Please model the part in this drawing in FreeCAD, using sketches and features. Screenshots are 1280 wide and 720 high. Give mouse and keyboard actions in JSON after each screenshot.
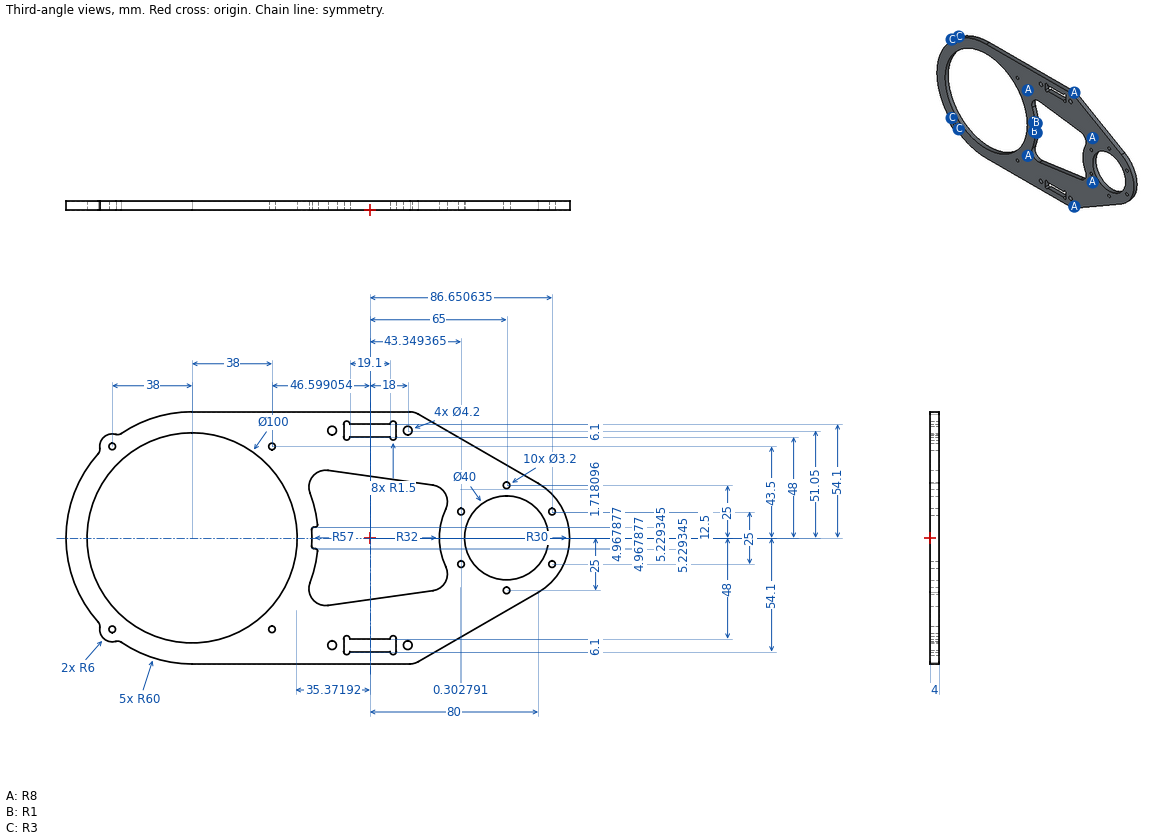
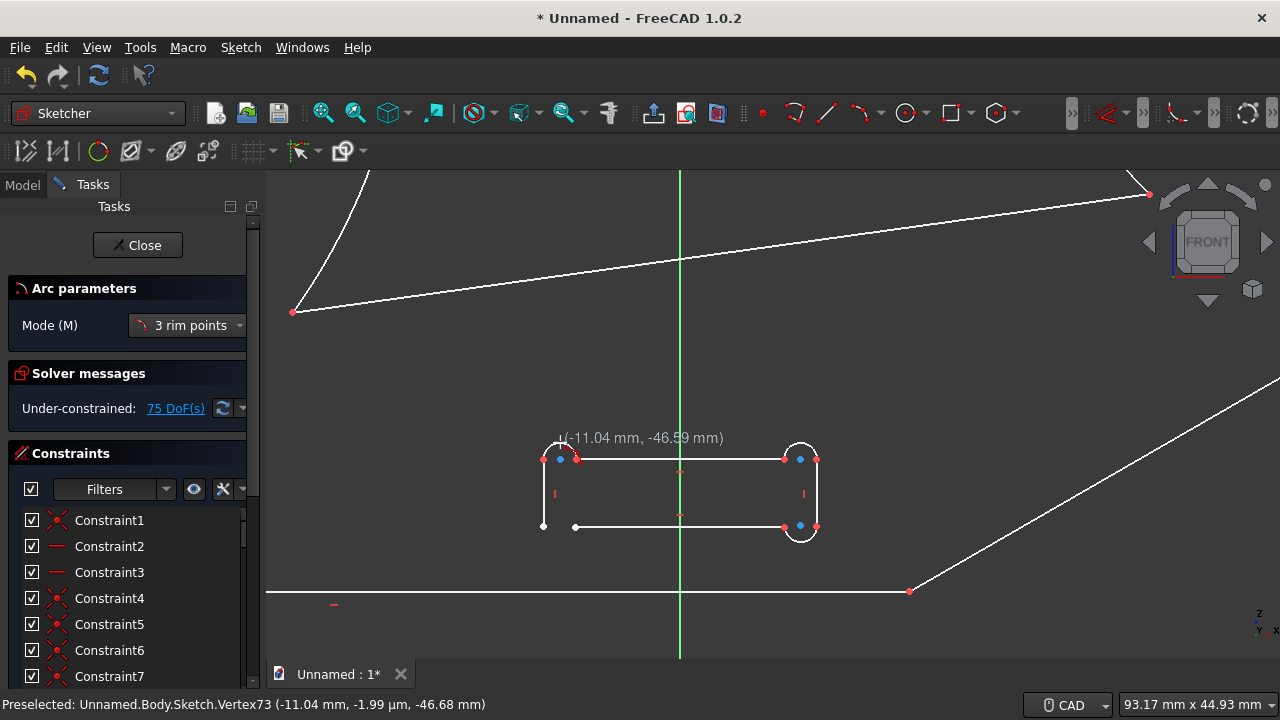
{"action": "left_click", "coordinate": [544, 527]}
{"action": "left_click", "coordinate": [576, 527]}
{"action": "left_click", "coordinate": [560, 541]}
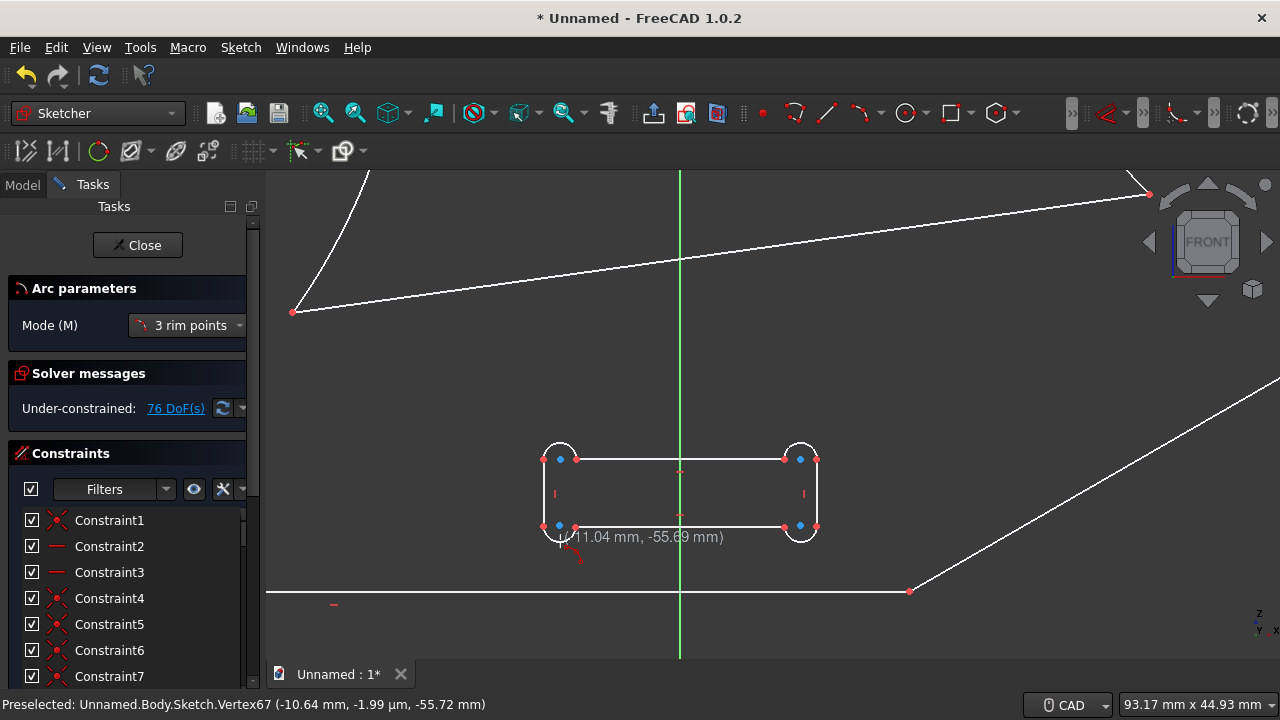
{"action": "left_click", "coordinate": [906, 114]}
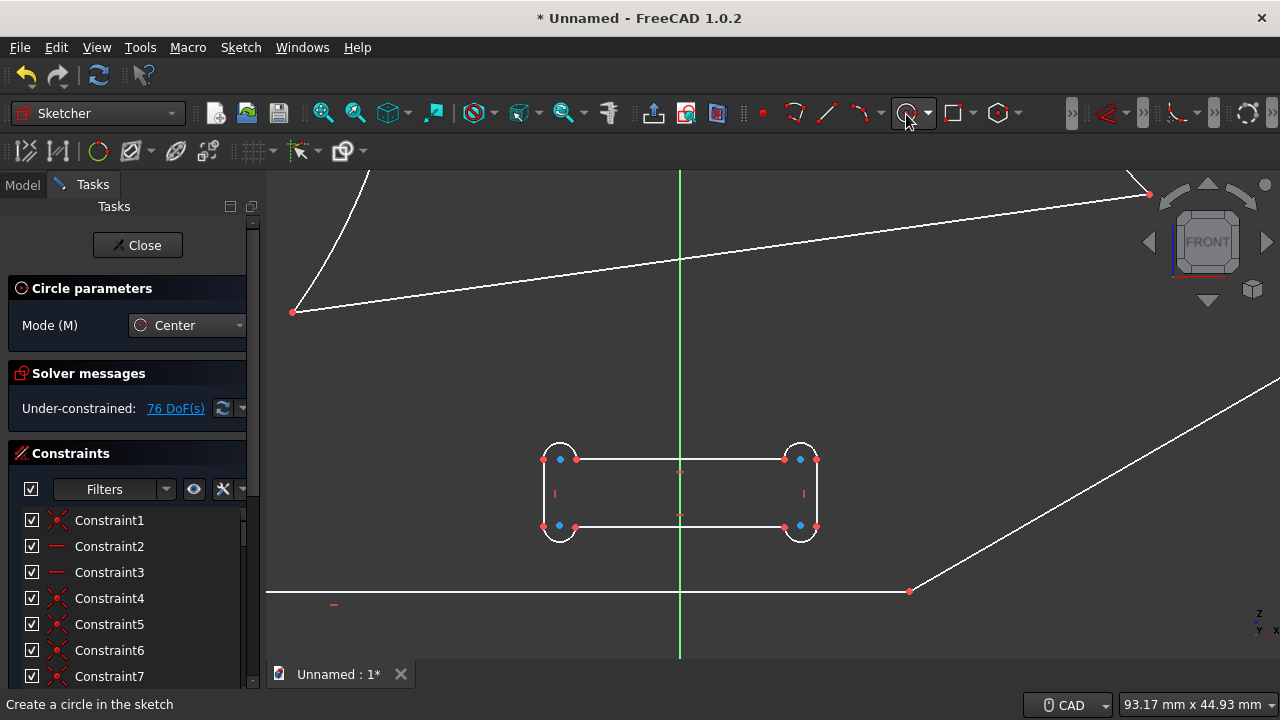
{"action": "scroll", "coordinate": [779, 536], "scroll_direction": "down", "scroll_amount": 8}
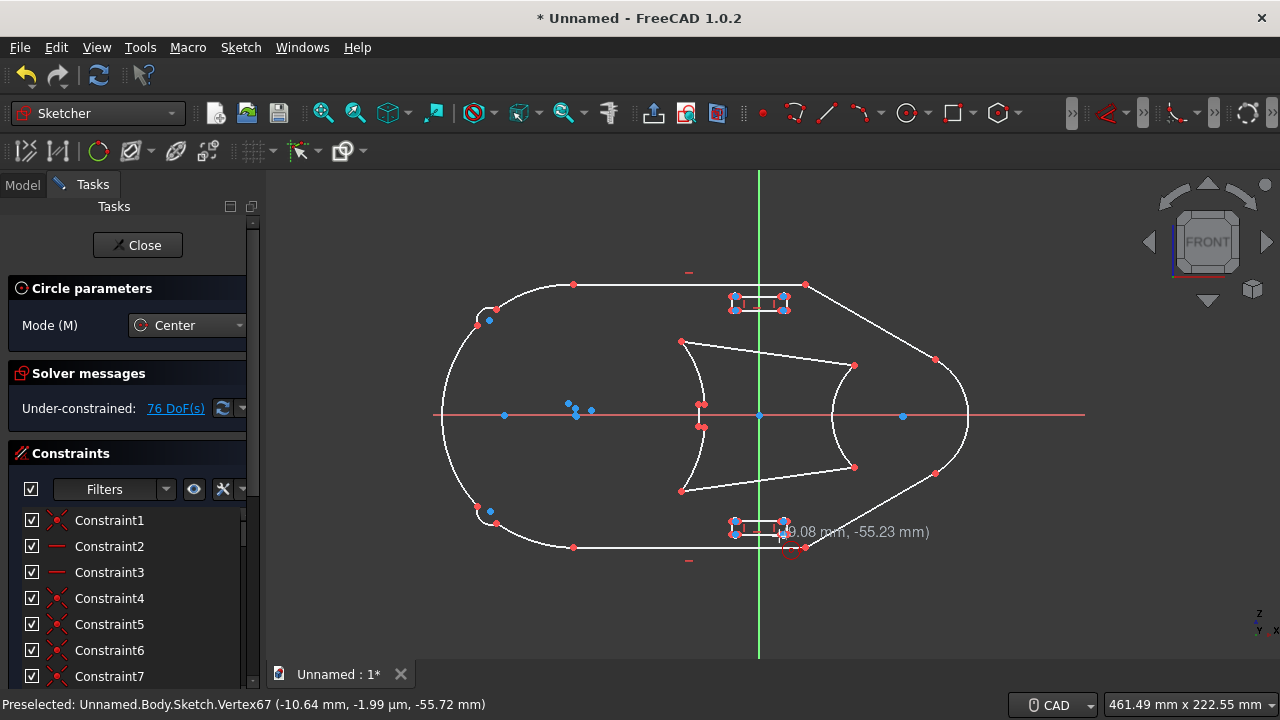
{"action": "scroll", "coordinate": [799, 303], "scroll_direction": "up", "scroll_amount": 8}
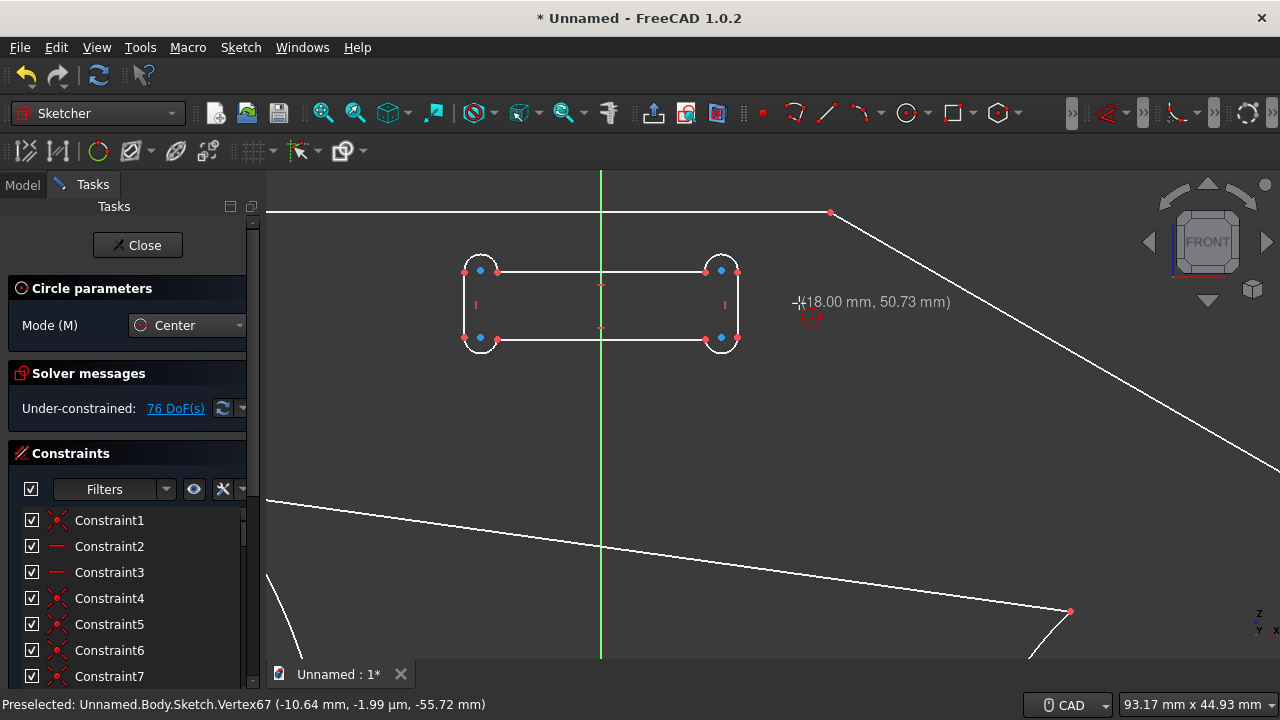
{"action": "scroll", "coordinate": [799, 302], "scroll_direction": "down", "scroll_amount": 8}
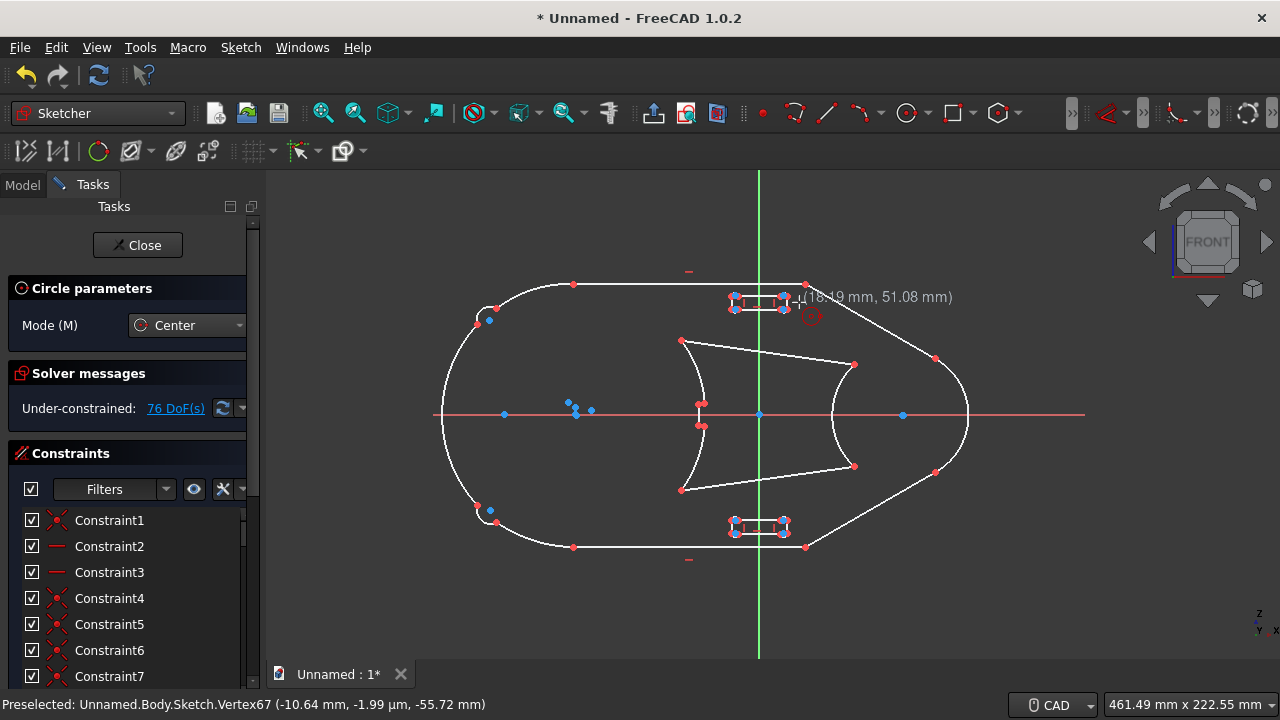
{"action": "scroll", "coordinate": [799, 302], "scroll_direction": "up", "scroll_amount": 2}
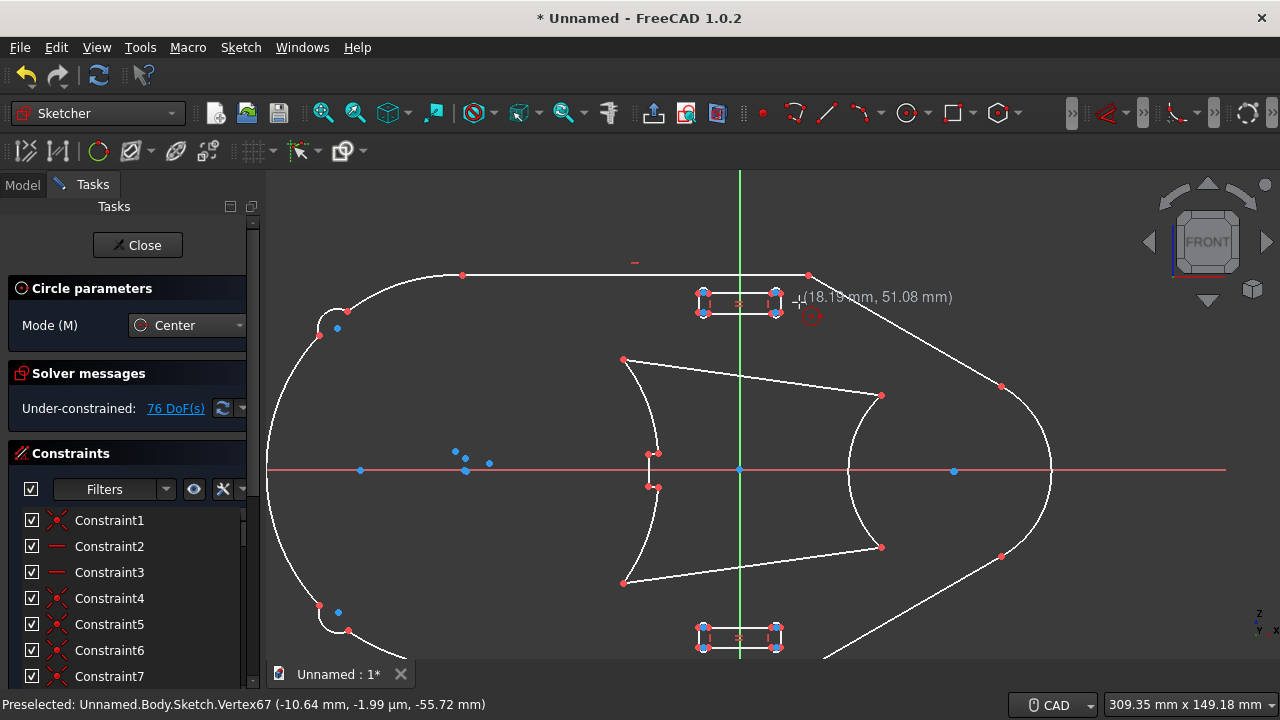
{"action": "left_click", "coordinate": [799, 303]}
{"action": "mouse_move", "coordinate": [804, 298]}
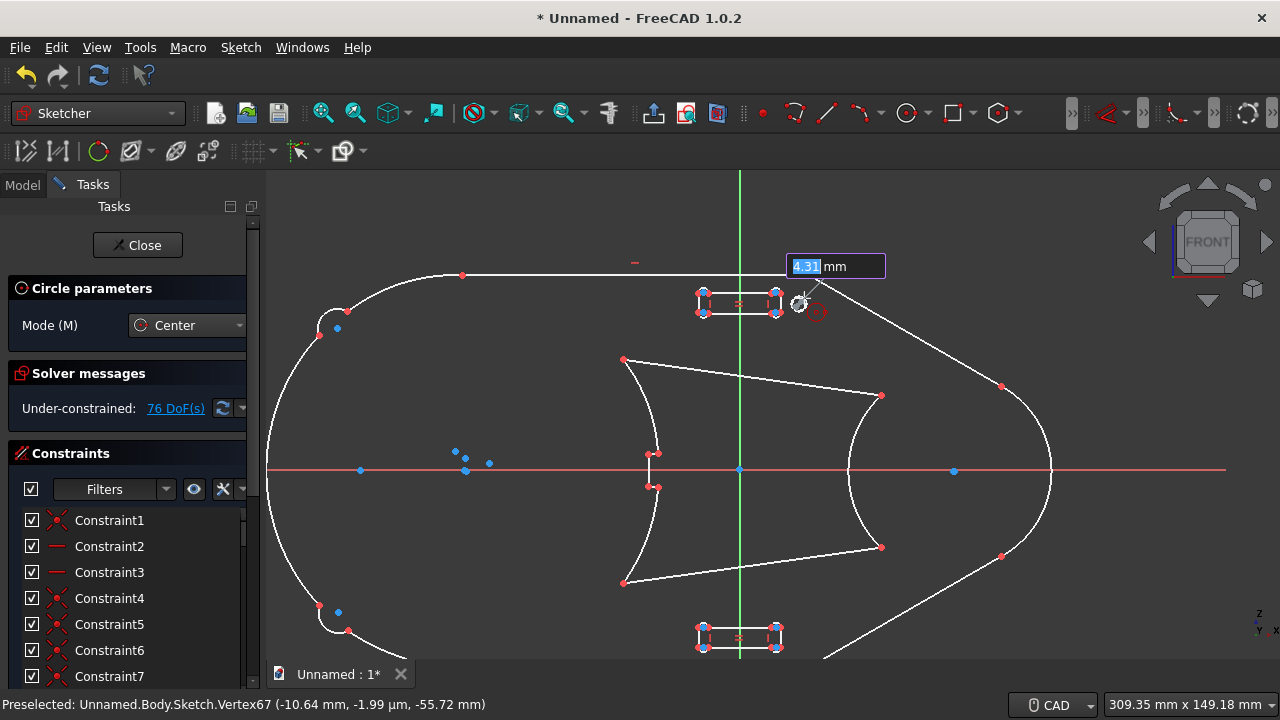
{"action": "type", "text": "4.2"}
{"action": "key", "text": "Return"}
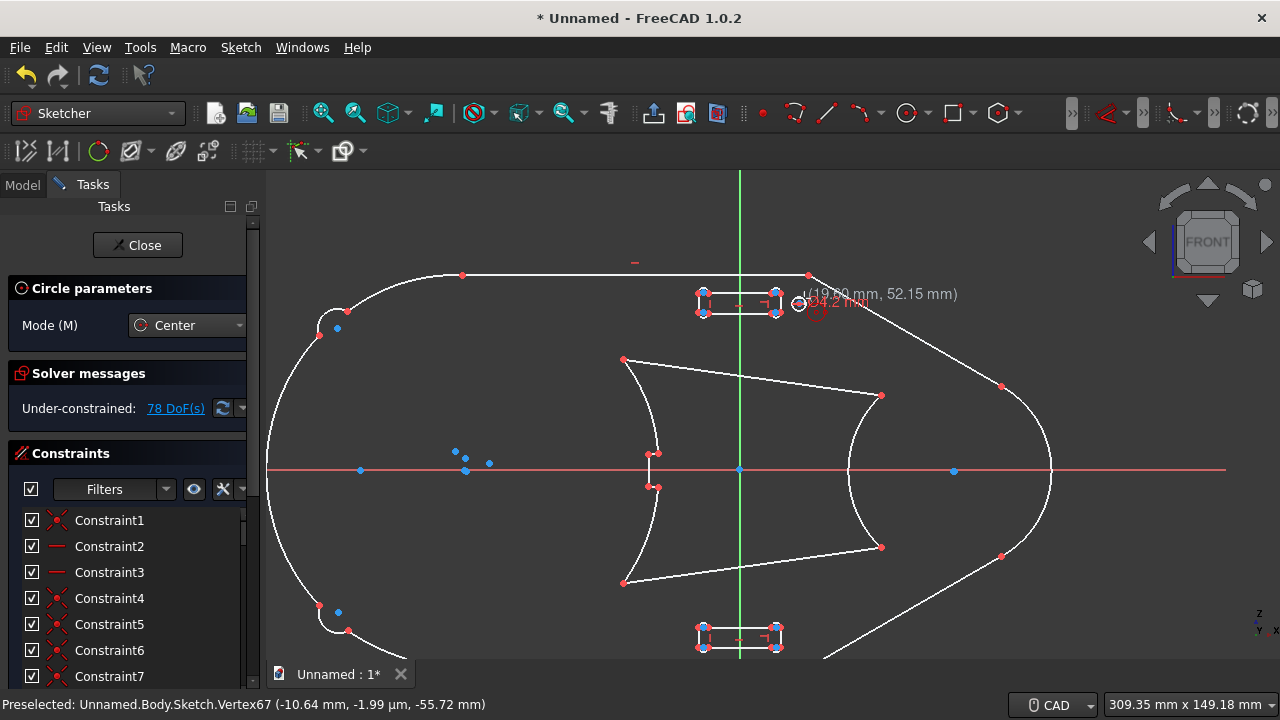
{"action": "scroll", "coordinate": [681, 303], "scroll_direction": "up", "scroll_amount": 6}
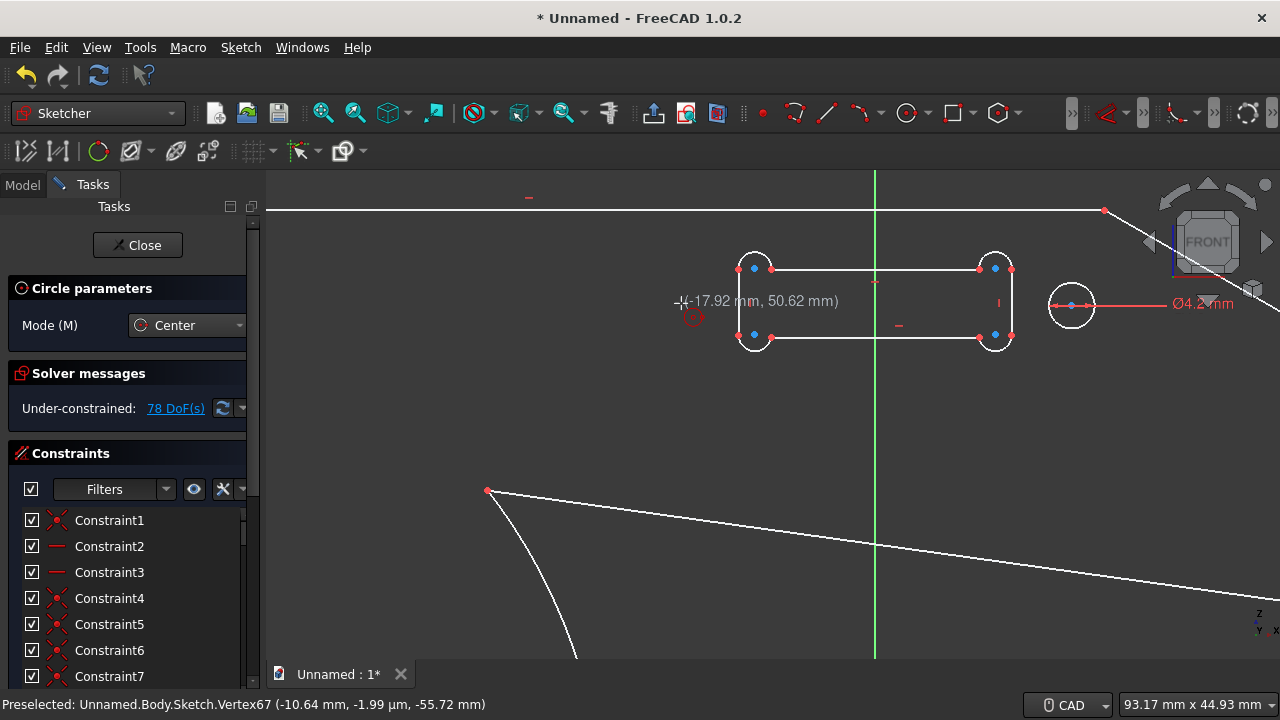
{"action": "scroll", "coordinate": [730, 303], "scroll_direction": "down", "scroll_amount": 8}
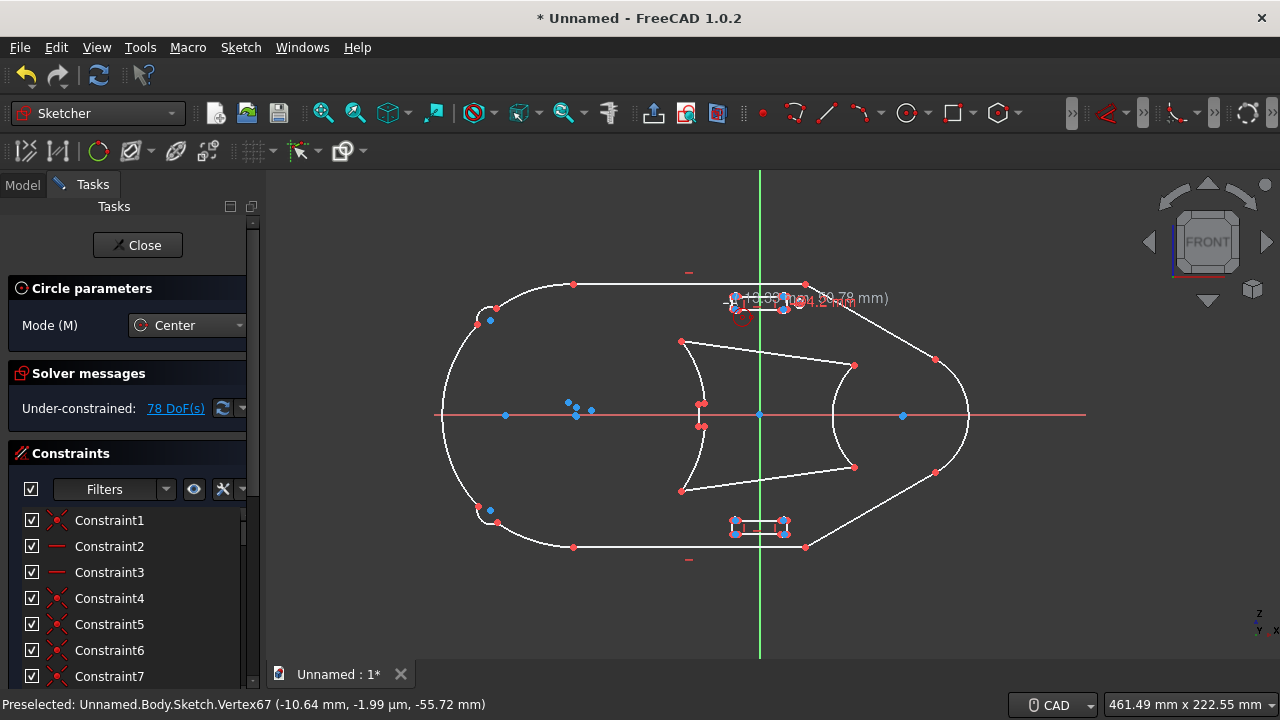
{"action": "scroll", "coordinate": [720, 303], "scroll_direction": "up", "scroll_amount": 2}